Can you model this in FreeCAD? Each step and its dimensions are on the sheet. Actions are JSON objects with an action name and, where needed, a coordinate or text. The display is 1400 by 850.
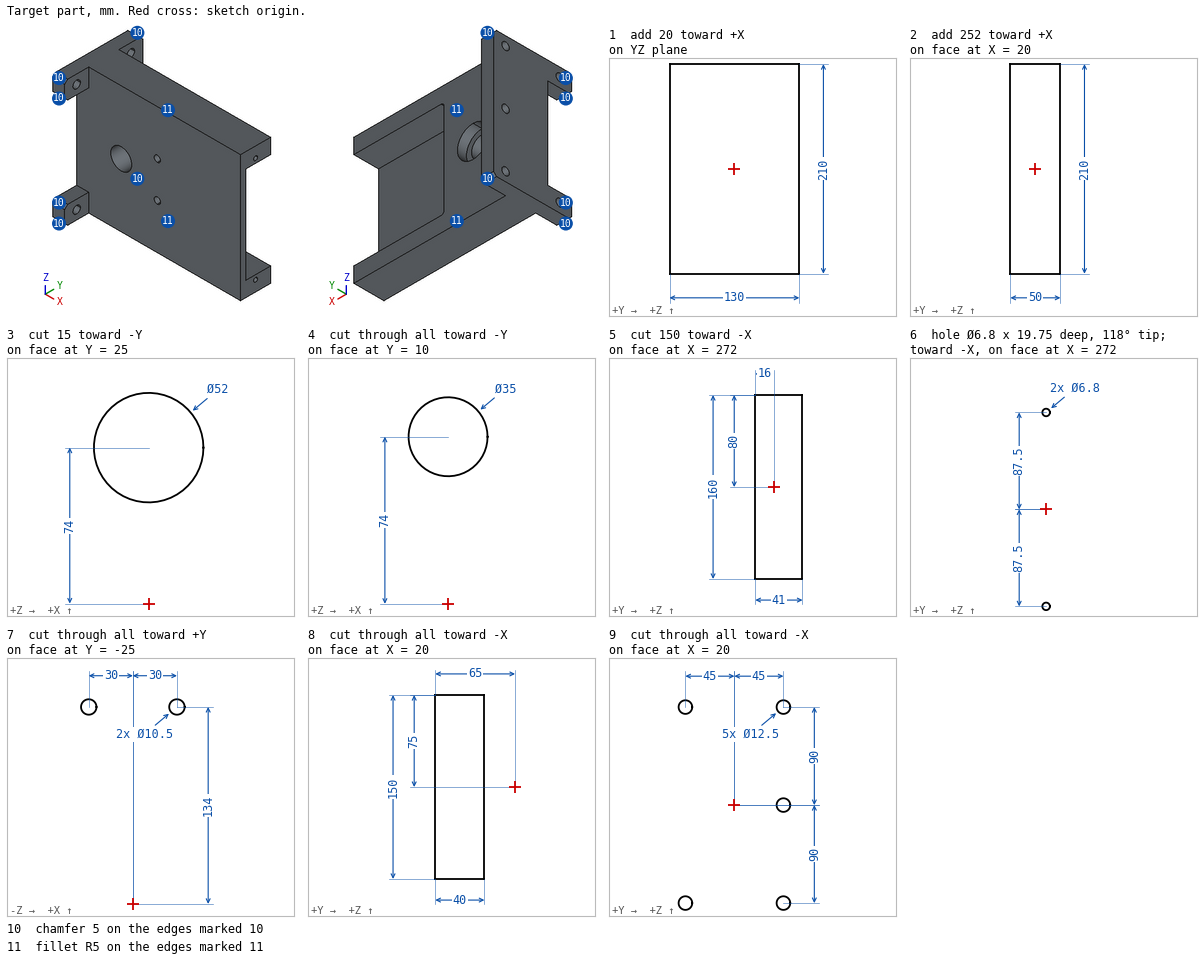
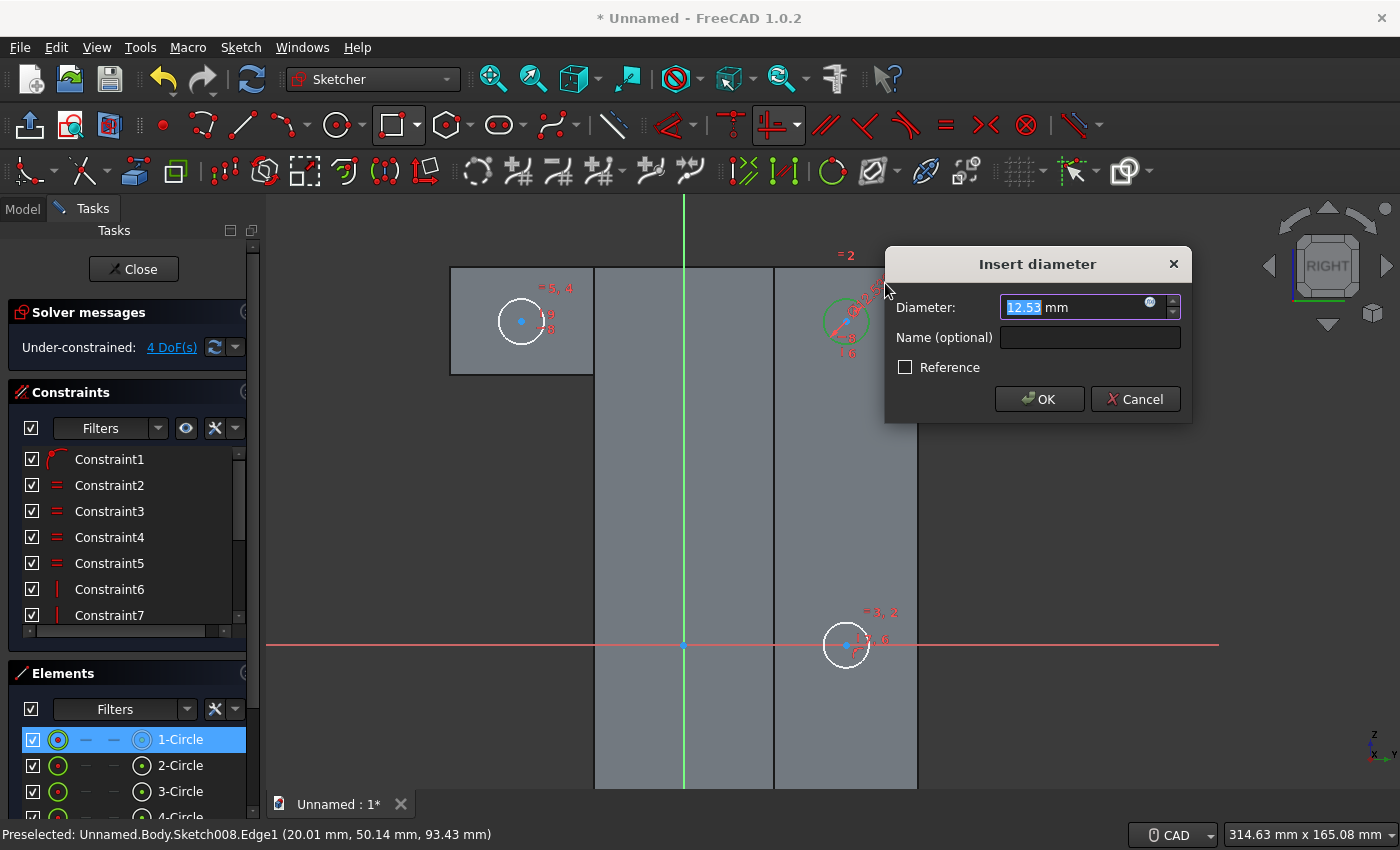
{"action": "type", "text": "12.5"}
{"action": "key", "text": "Return"}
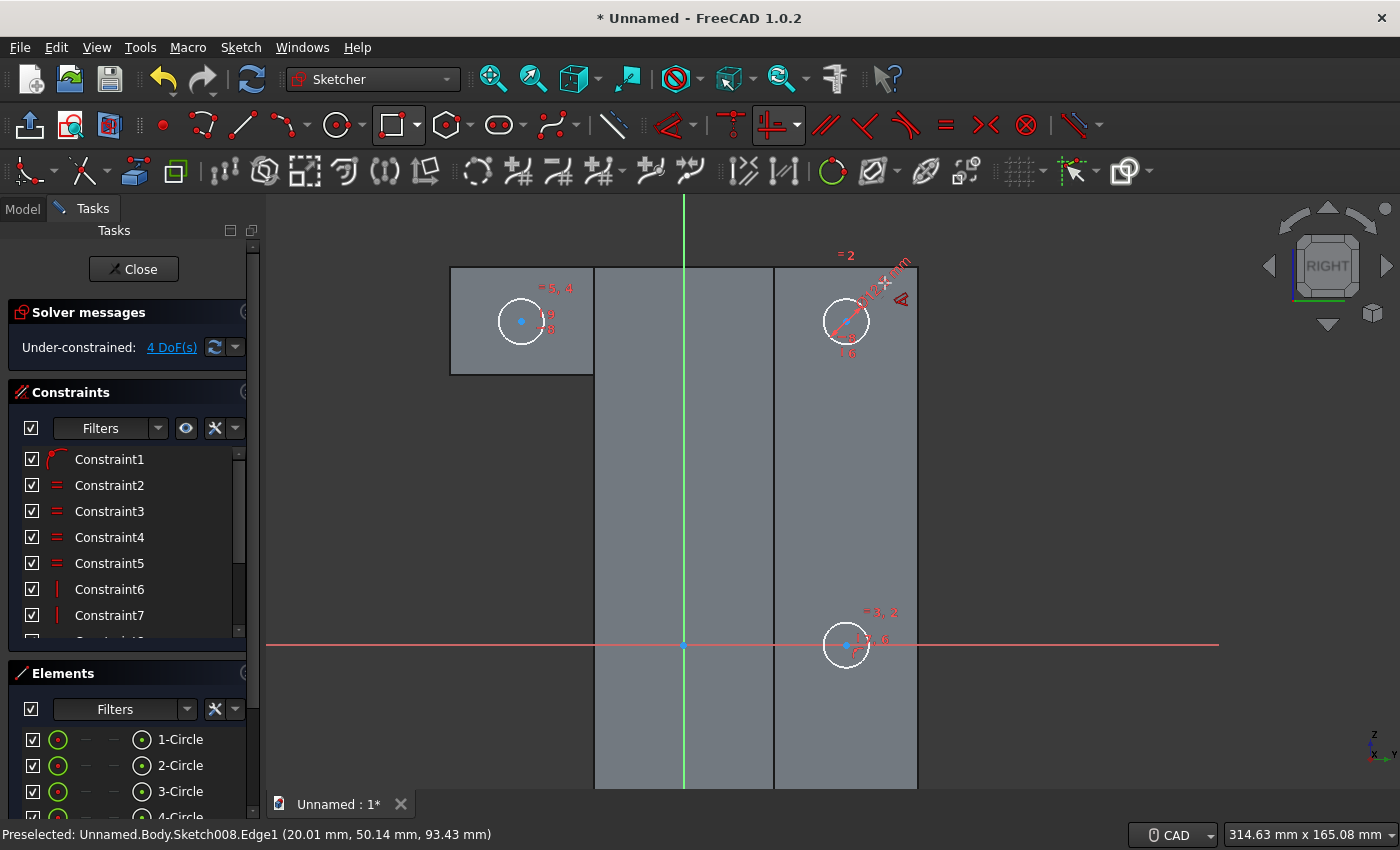
{"action": "left_click", "coordinate": [846, 322]}
{"action": "left_click", "coordinate": [765, 288]}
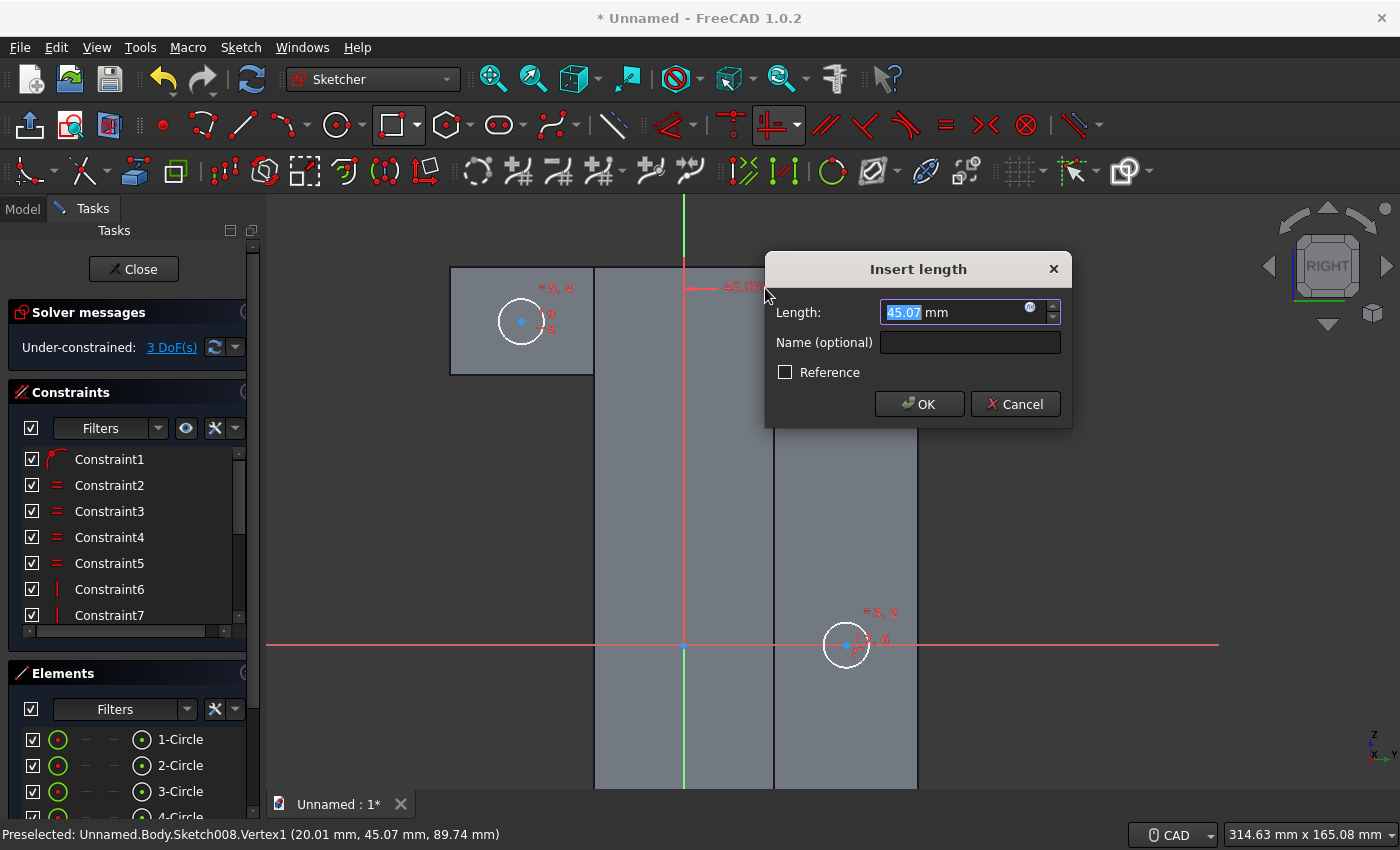
{"action": "type", "text": "45"}
{"action": "key", "text": "Return"}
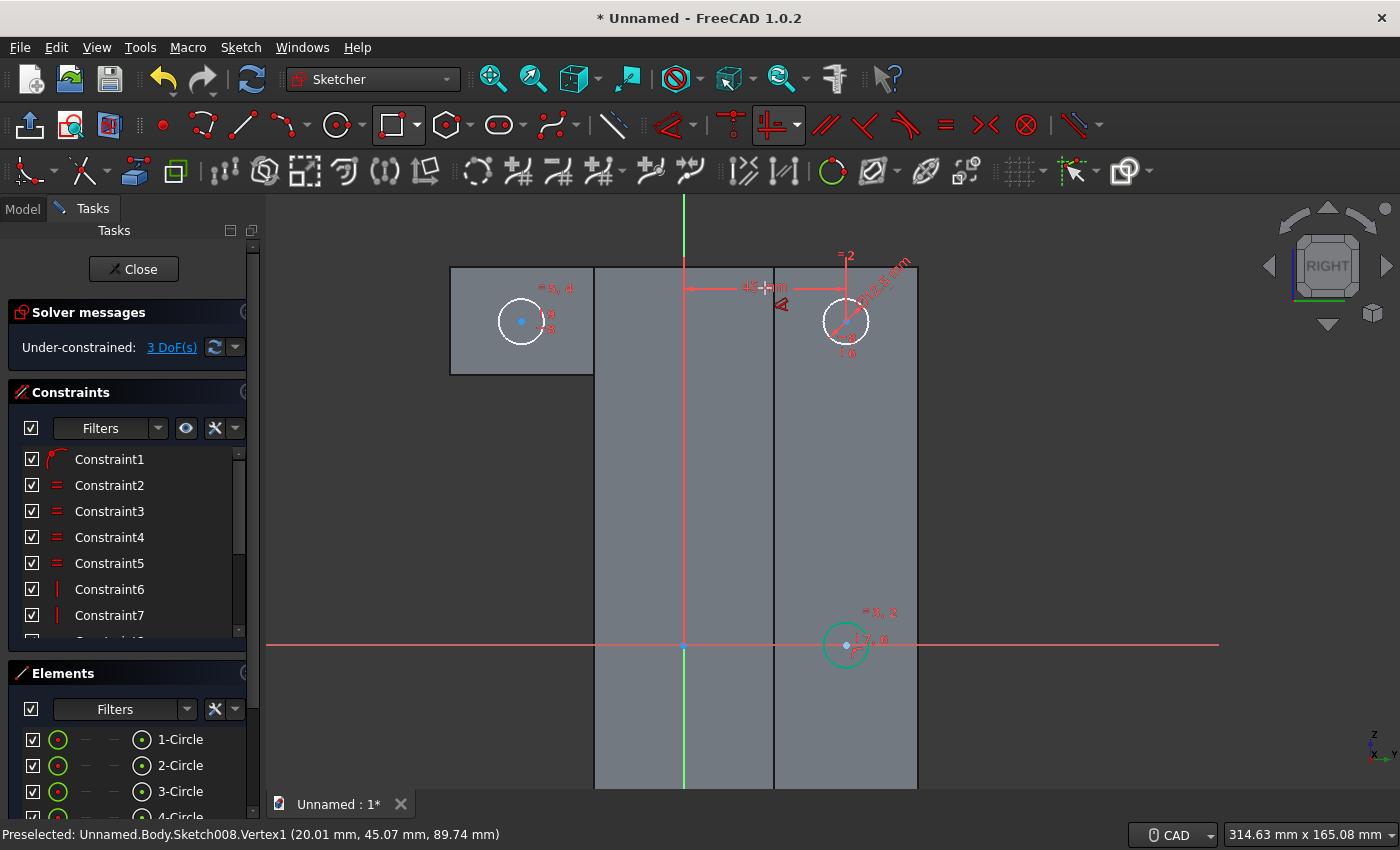
{"action": "left_click", "coordinate": [846, 322]}
{"action": "left_click", "coordinate": [880, 483]}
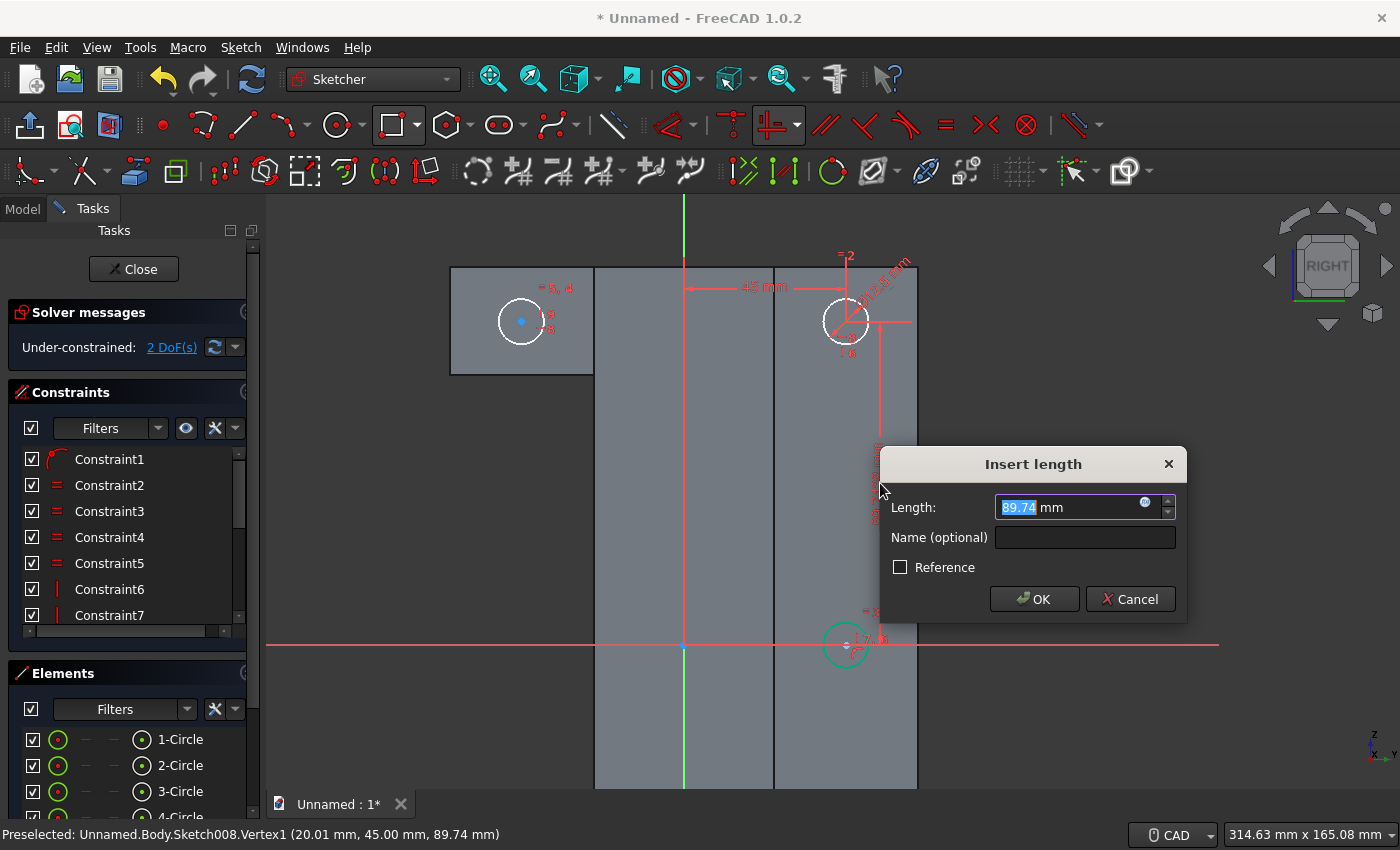
{"action": "type", "text": "90"}
{"action": "key", "text": "Return"}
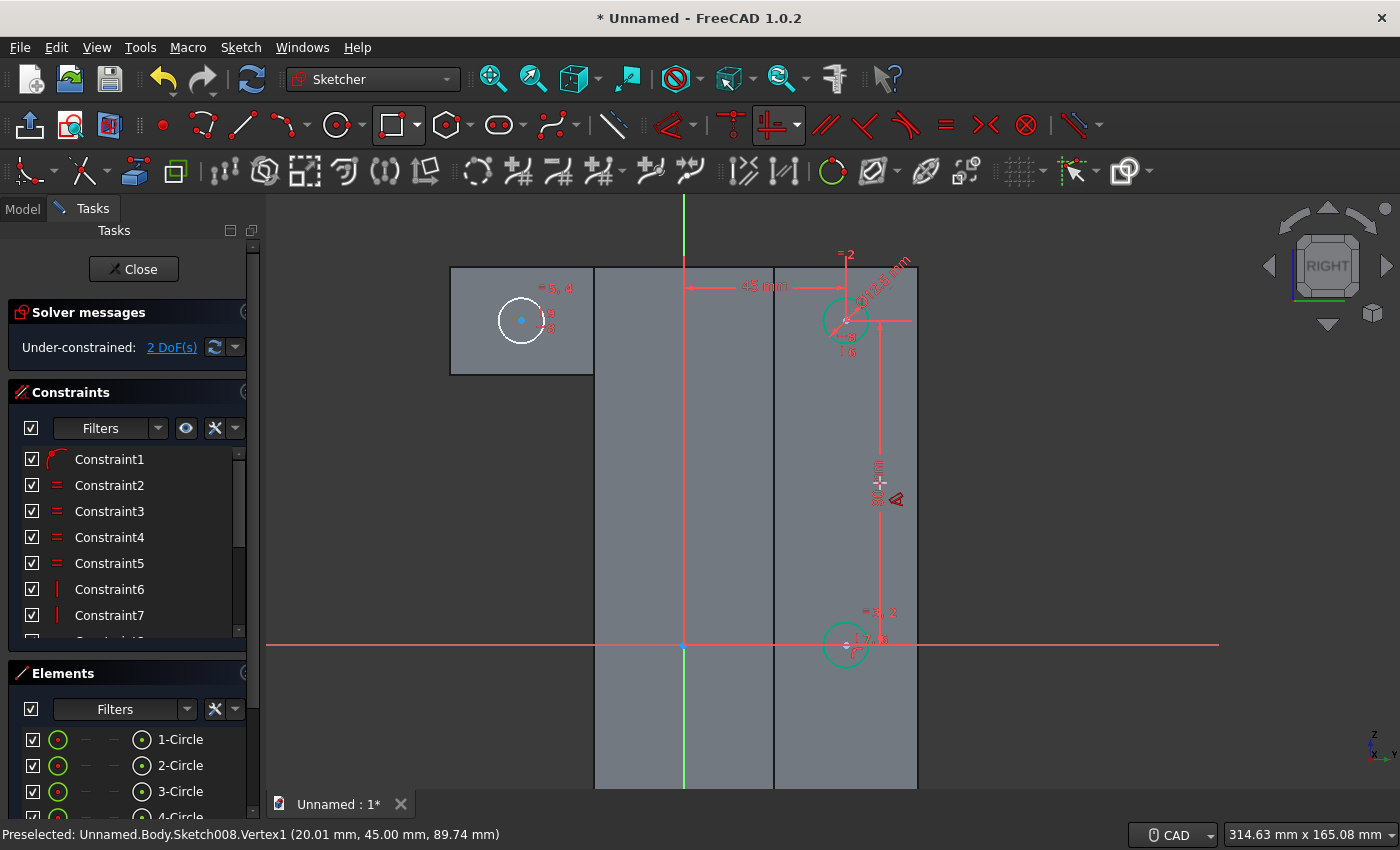
{"action": "scroll", "coordinate": [863, 305], "scroll_direction": "down", "scroll_amount": 3}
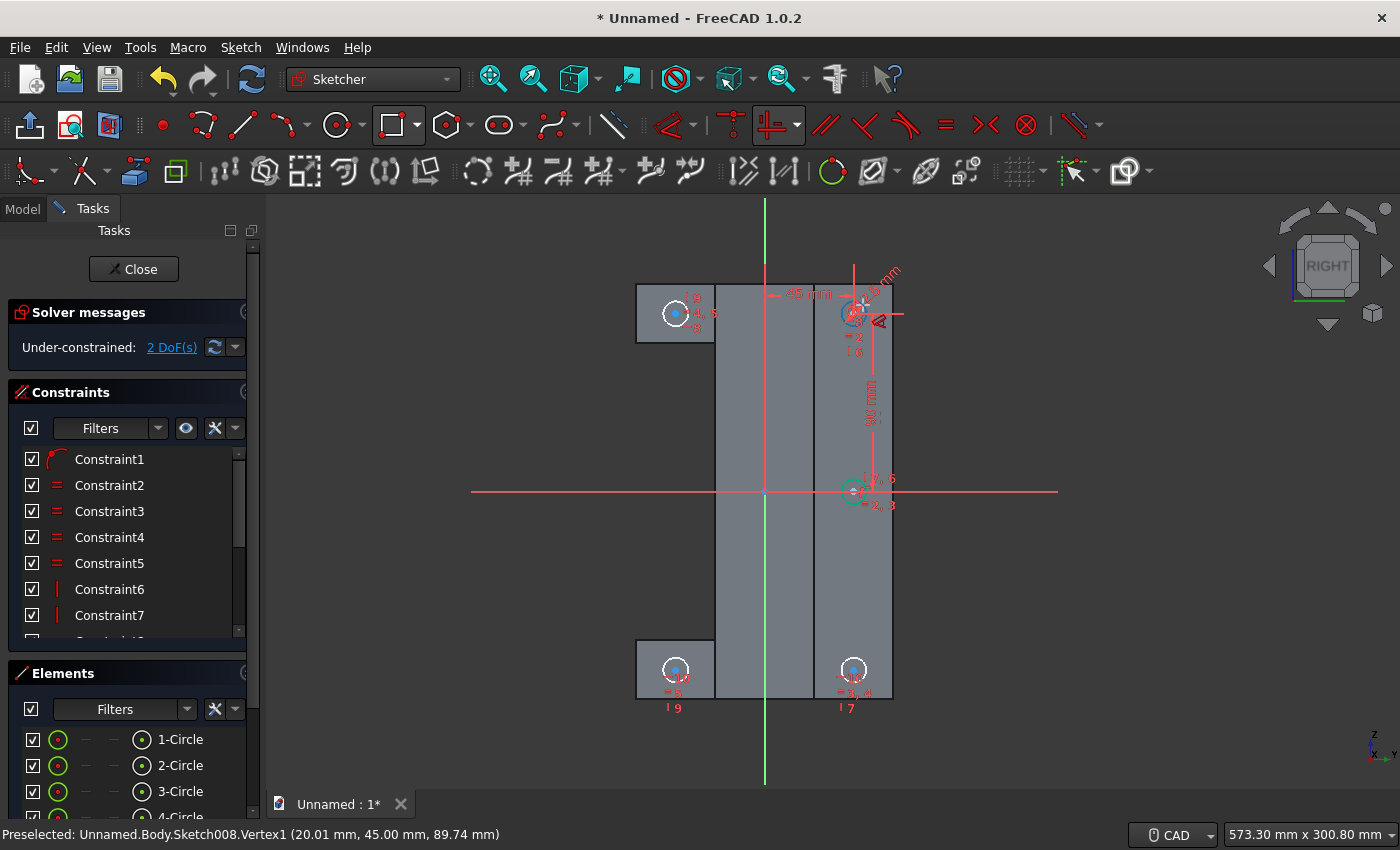
{"action": "left_click", "coordinate": [854, 670]}
{"action": "left_click", "coordinate": [888, 581]}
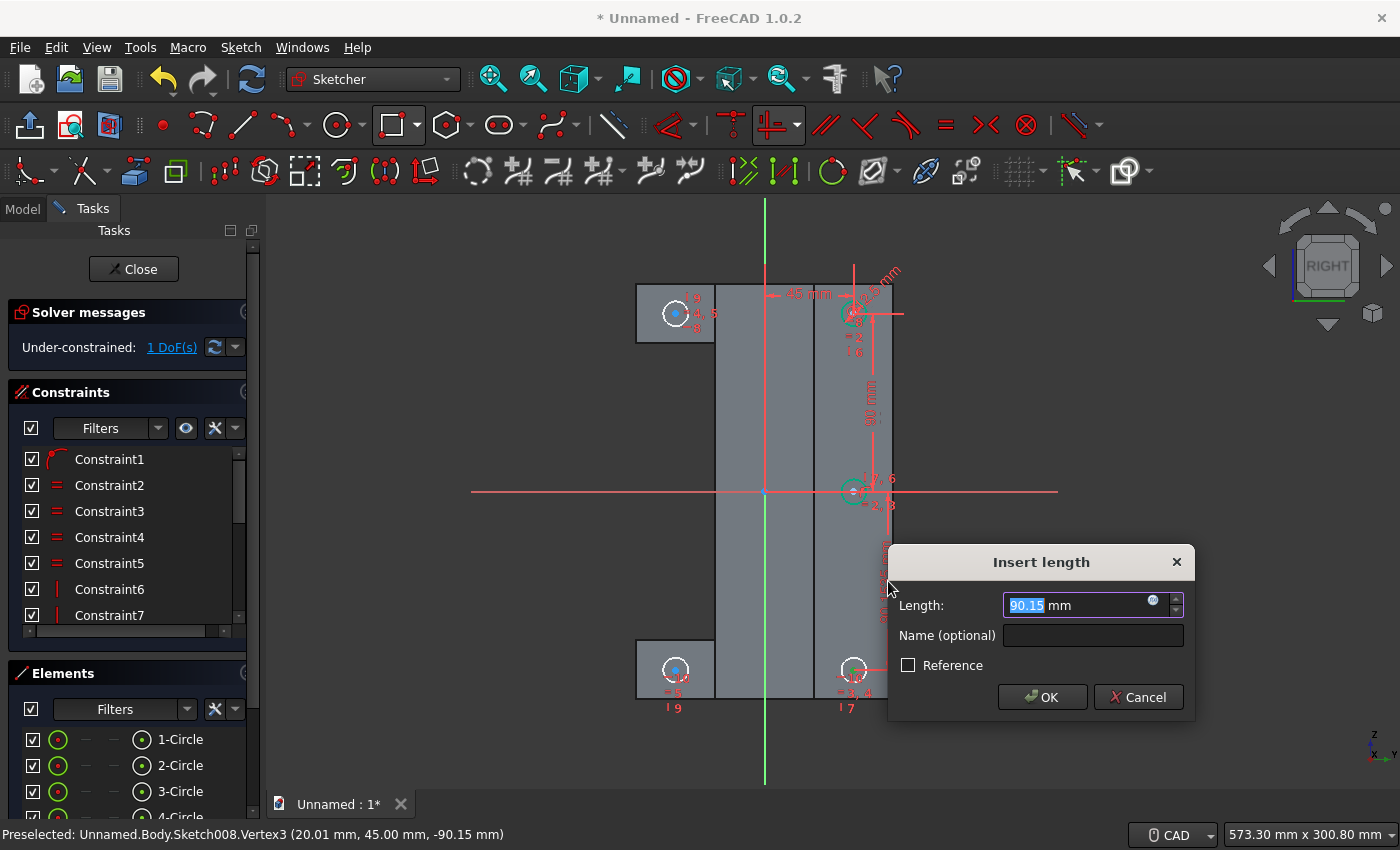
{"action": "type", "text": "90"}
{"action": "key", "text": "Return"}